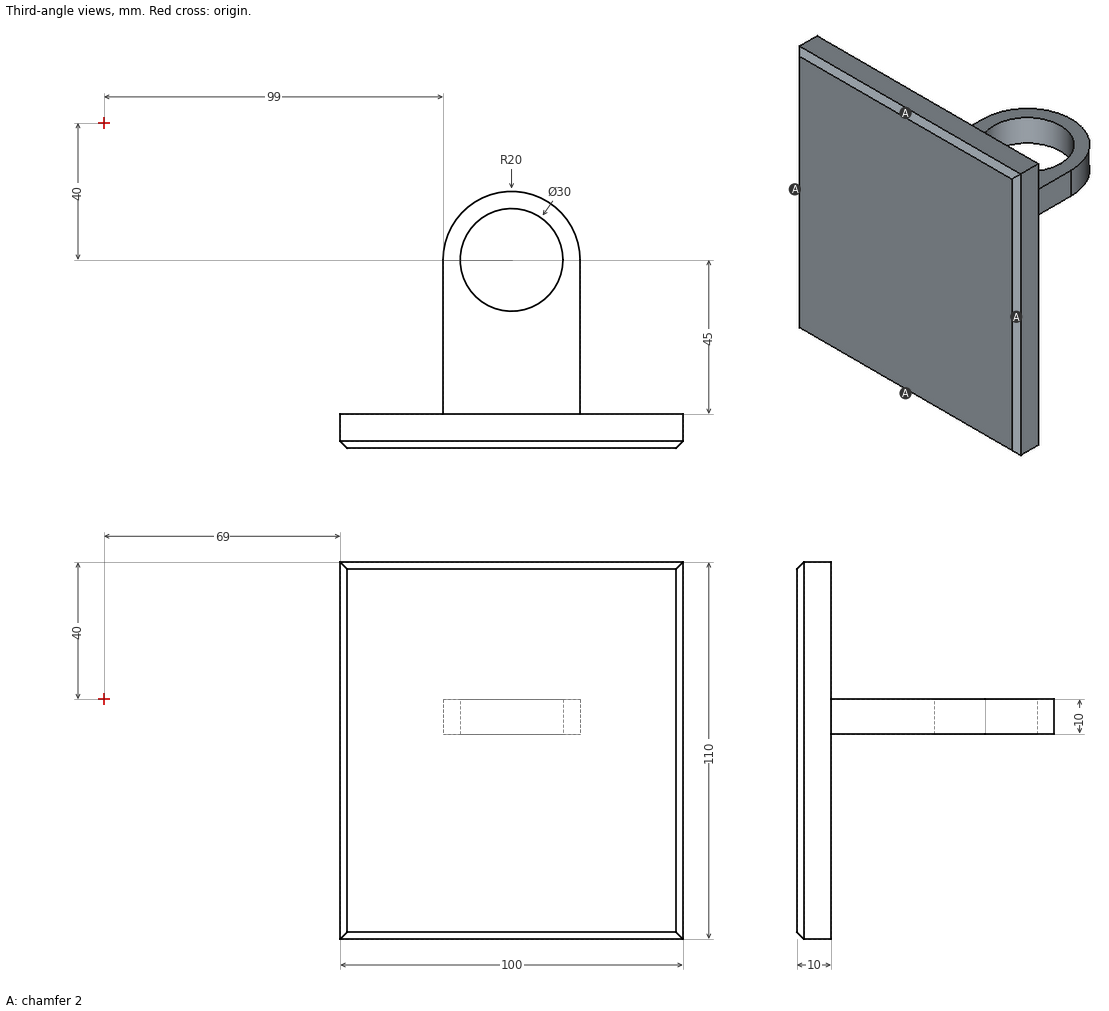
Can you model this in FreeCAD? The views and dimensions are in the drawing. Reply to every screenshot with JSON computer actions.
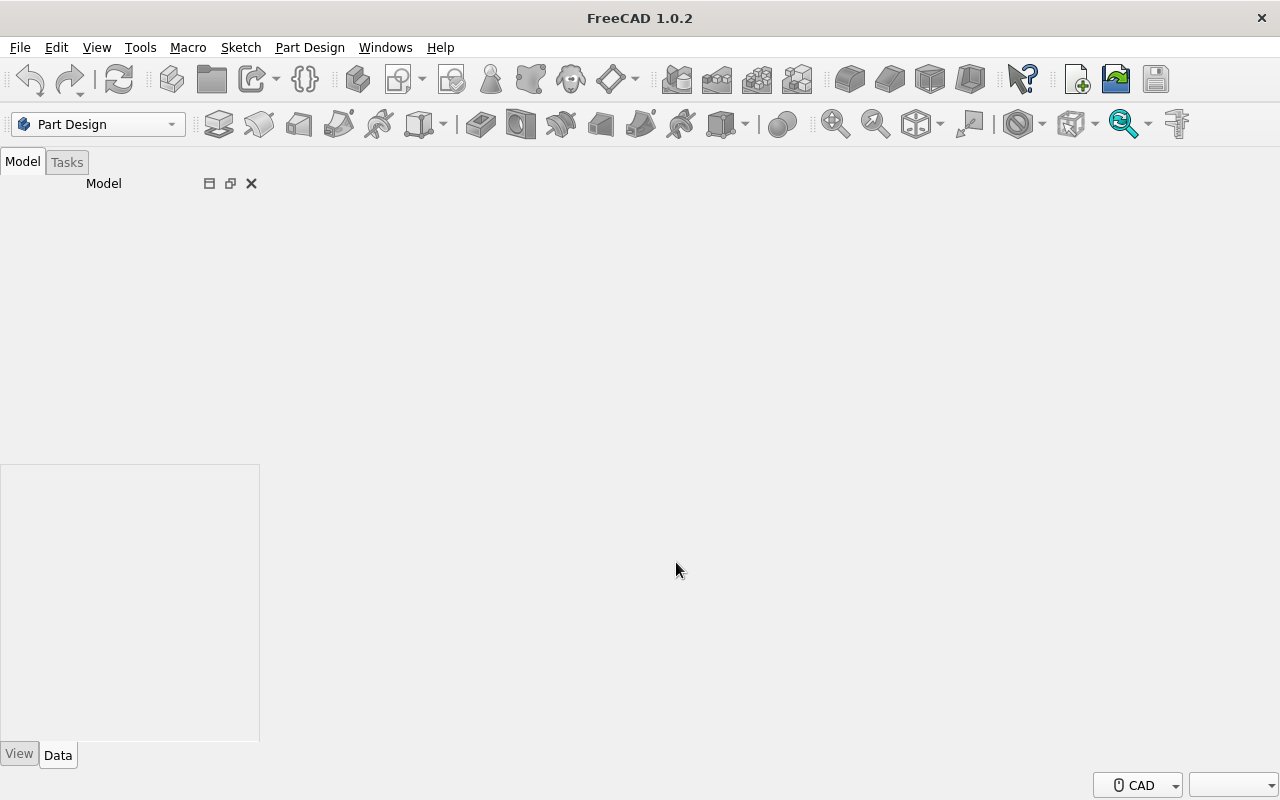
{"action": "left_click", "coordinate": [1076, 80]}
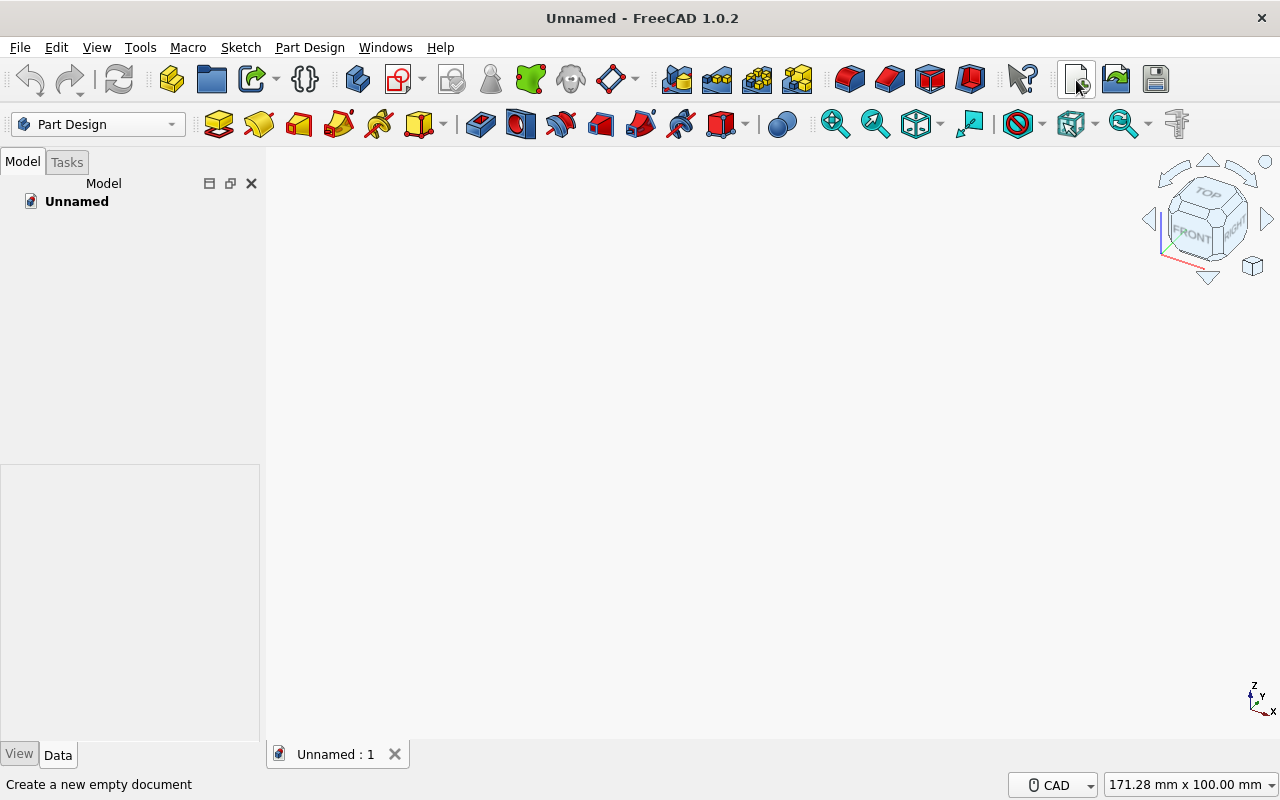
{"action": "left_click", "coordinate": [398, 80]}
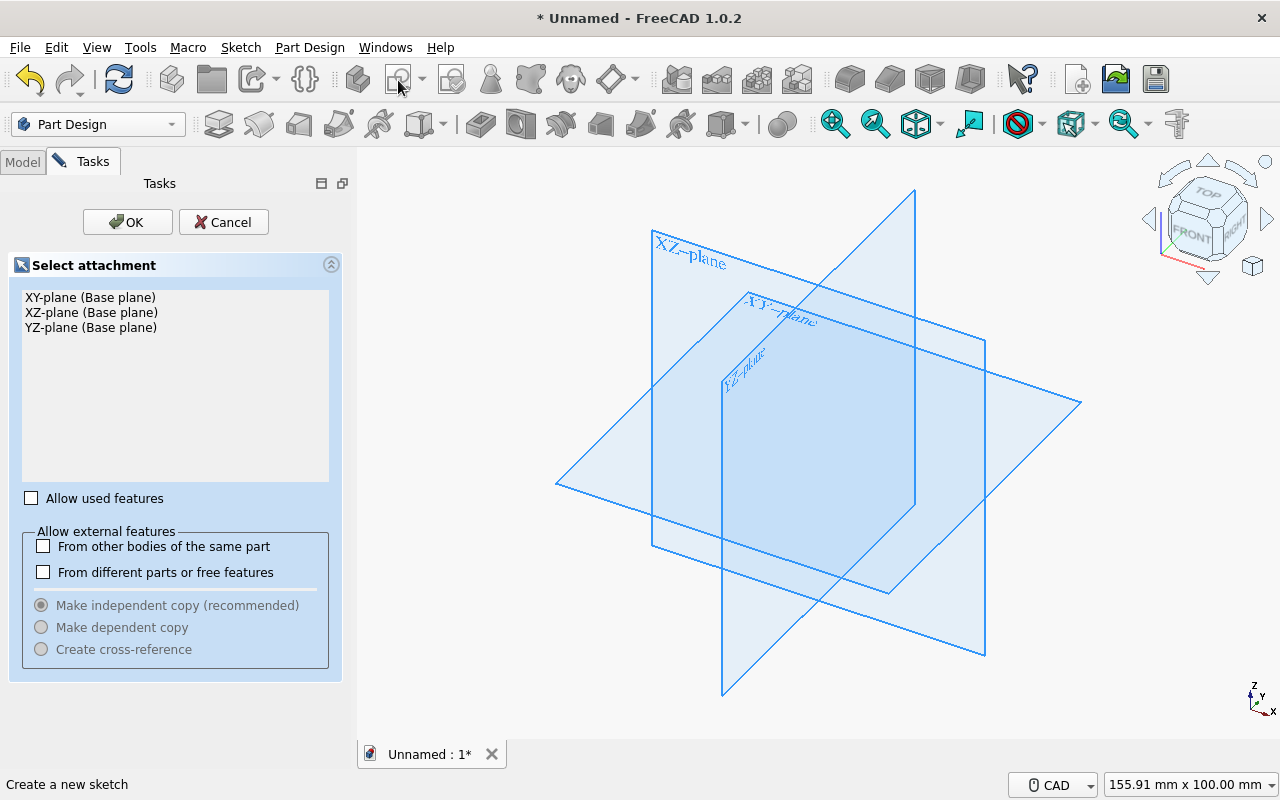
{"action": "left_click", "coordinate": [82, 298]}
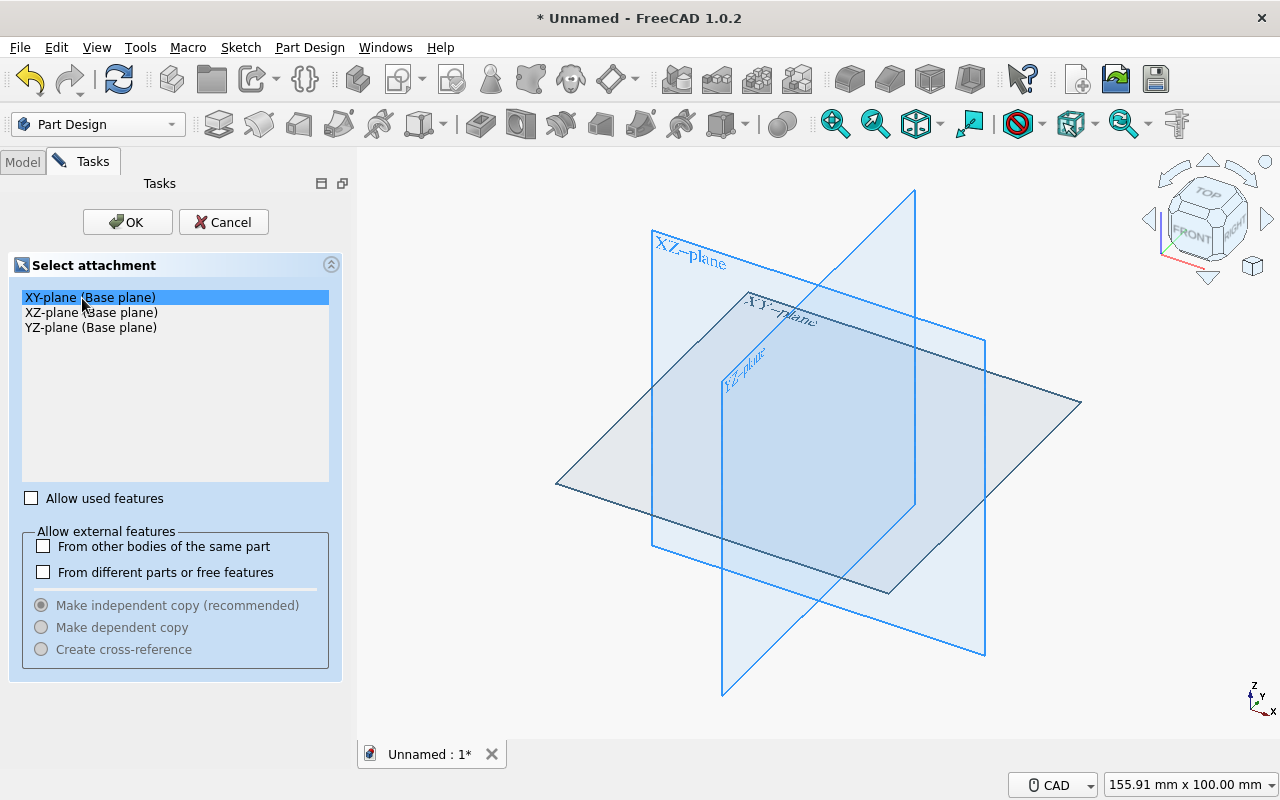
{"action": "left_click", "coordinate": [128, 222]}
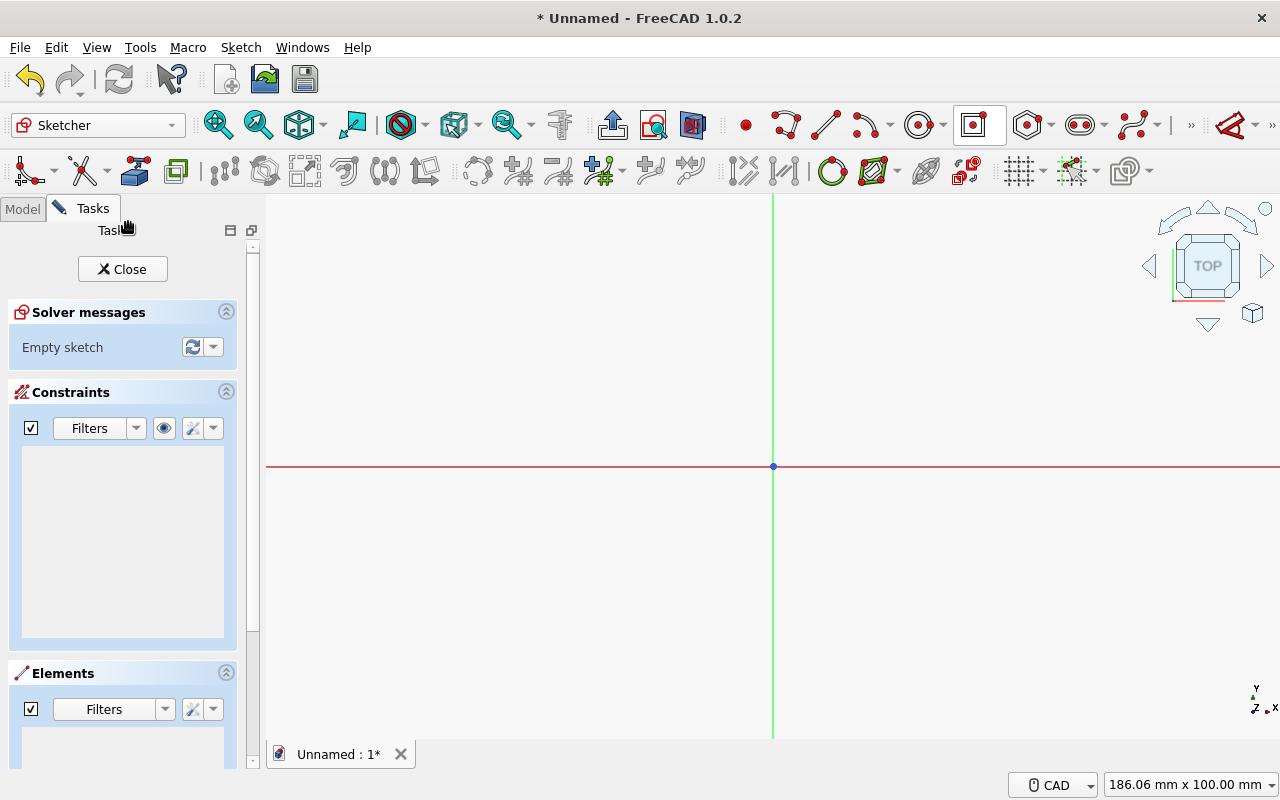
{"action": "scroll", "coordinate": [294, 222], "scroll_direction": "down", "scroll_amount": 3}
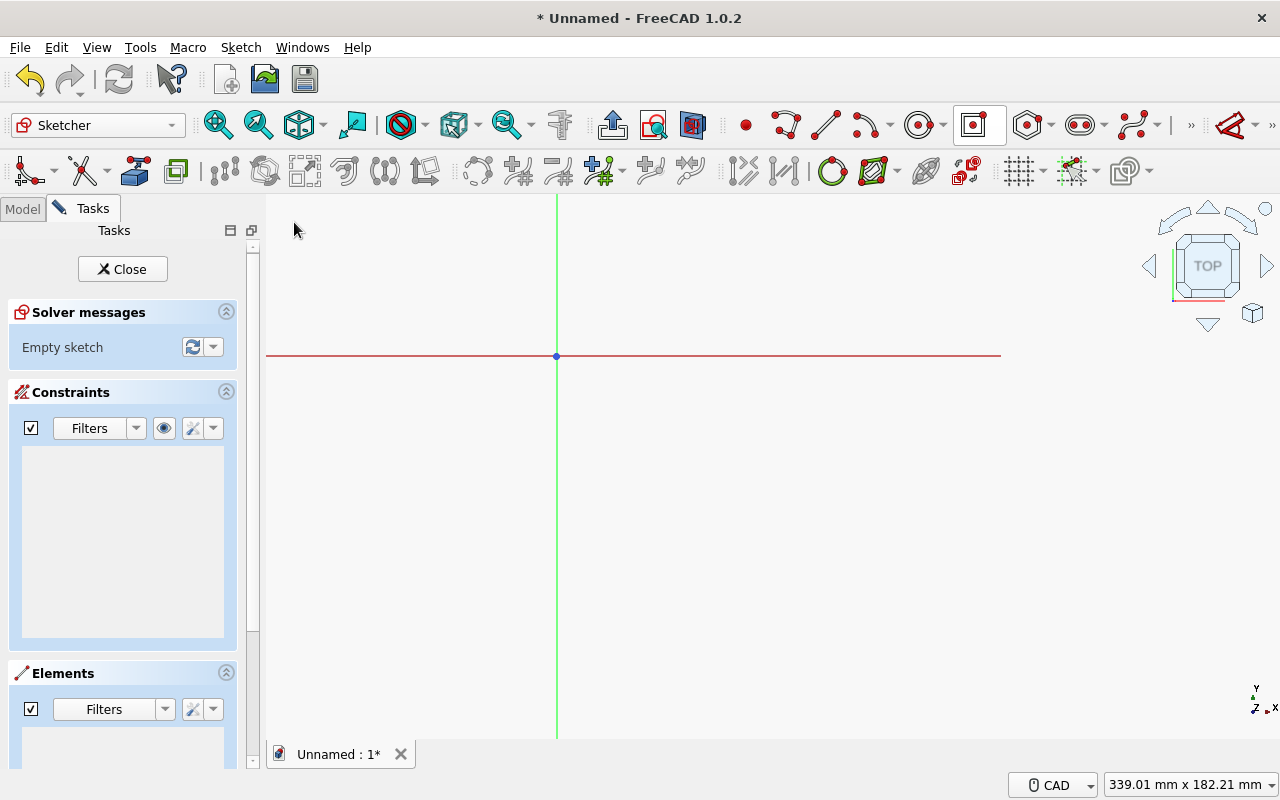
{"action": "scroll", "coordinate": [887, 518], "scroll_direction": "up", "scroll_amount": 2}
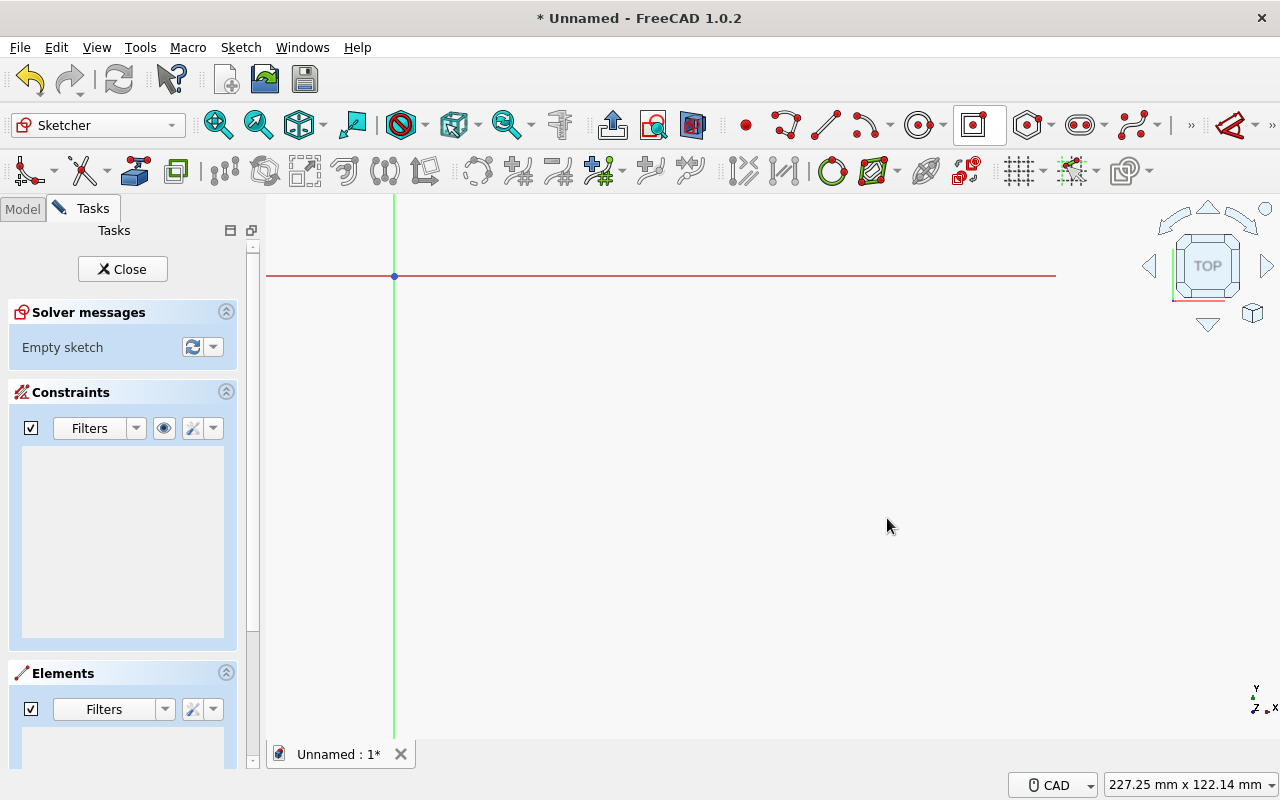
{"action": "left_click", "coordinate": [786, 126]}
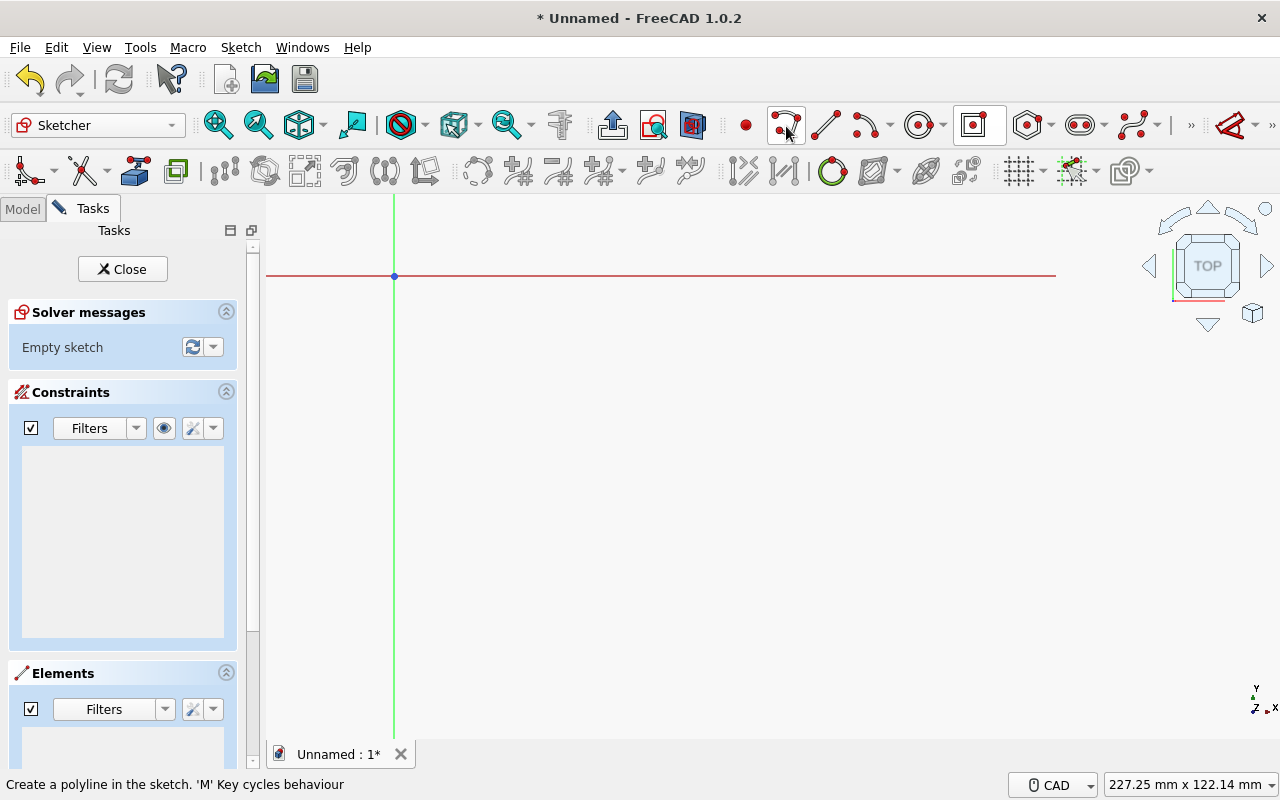
{"action": "left_click", "coordinate": [836, 455]}
{"action": "left_click", "coordinate": [836, 656]}
{"action": "left_click", "coordinate": [1014, 656]}
{"action": "left_click", "coordinate": [1014, 455]}
{"action": "right_click", "coordinate": [1014, 455]}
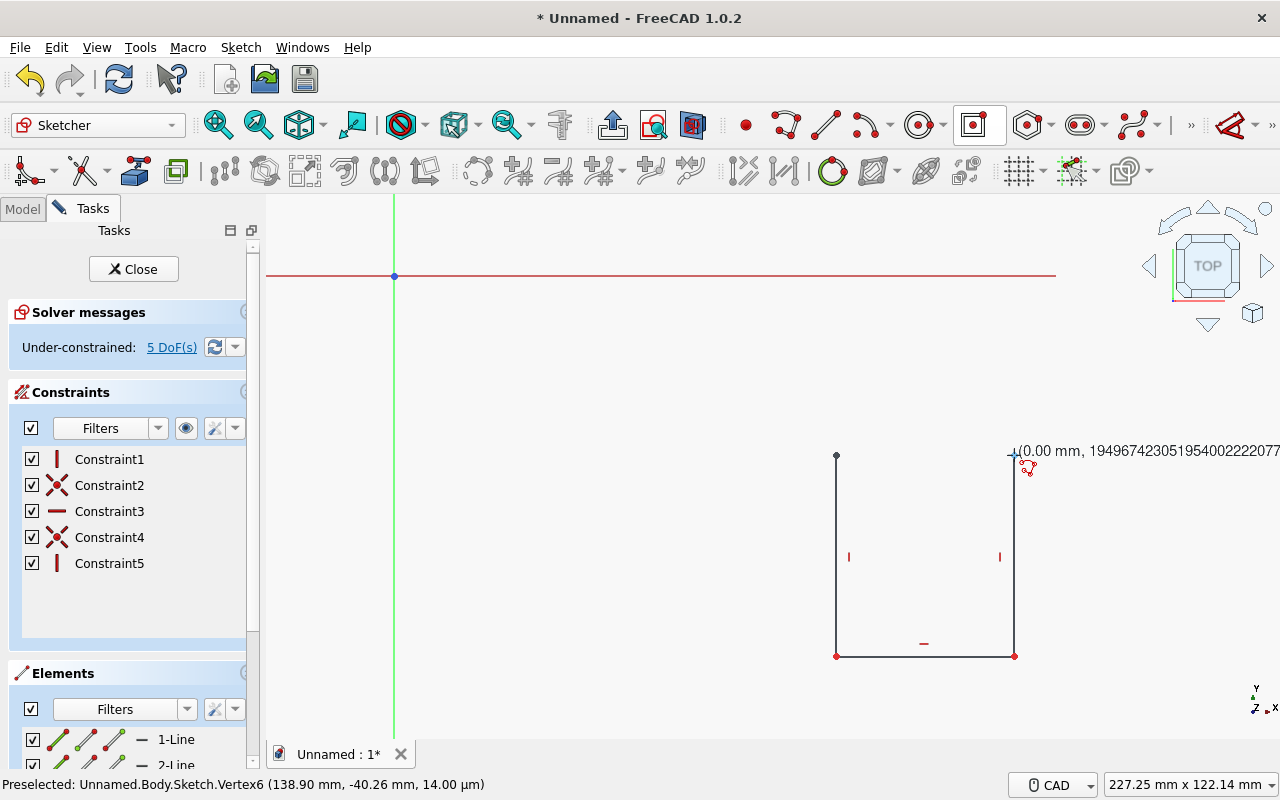
{"action": "key", "text": "g 3 a"}